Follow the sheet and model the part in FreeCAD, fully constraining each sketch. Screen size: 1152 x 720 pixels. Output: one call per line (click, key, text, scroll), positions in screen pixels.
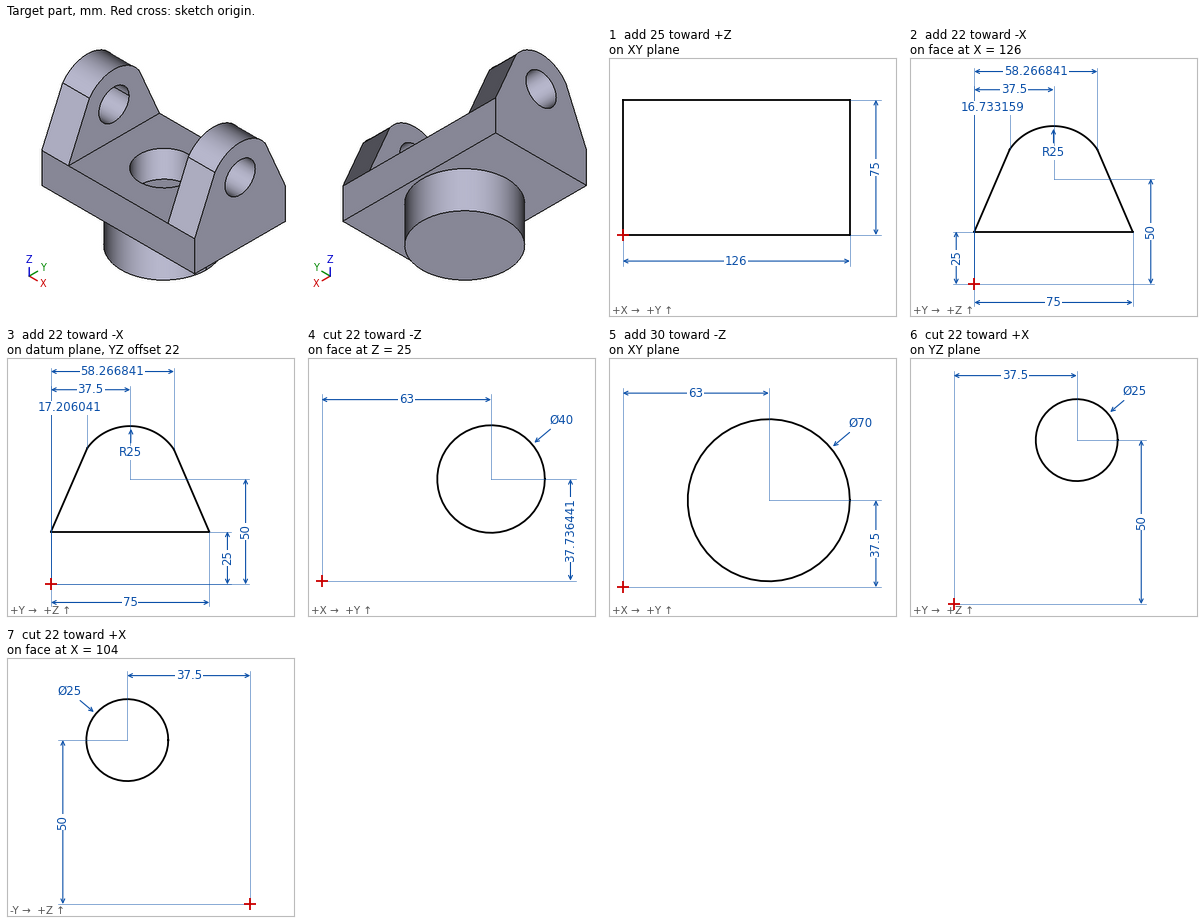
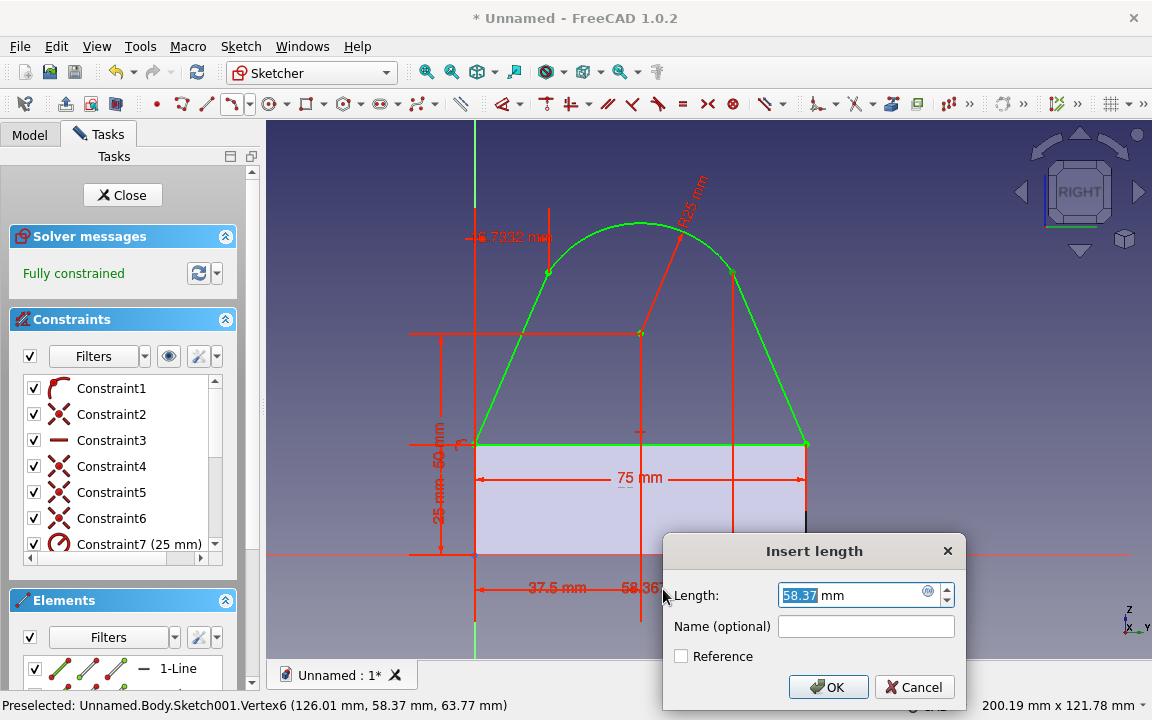
text(58.266841)
key(Return)
key(Escape)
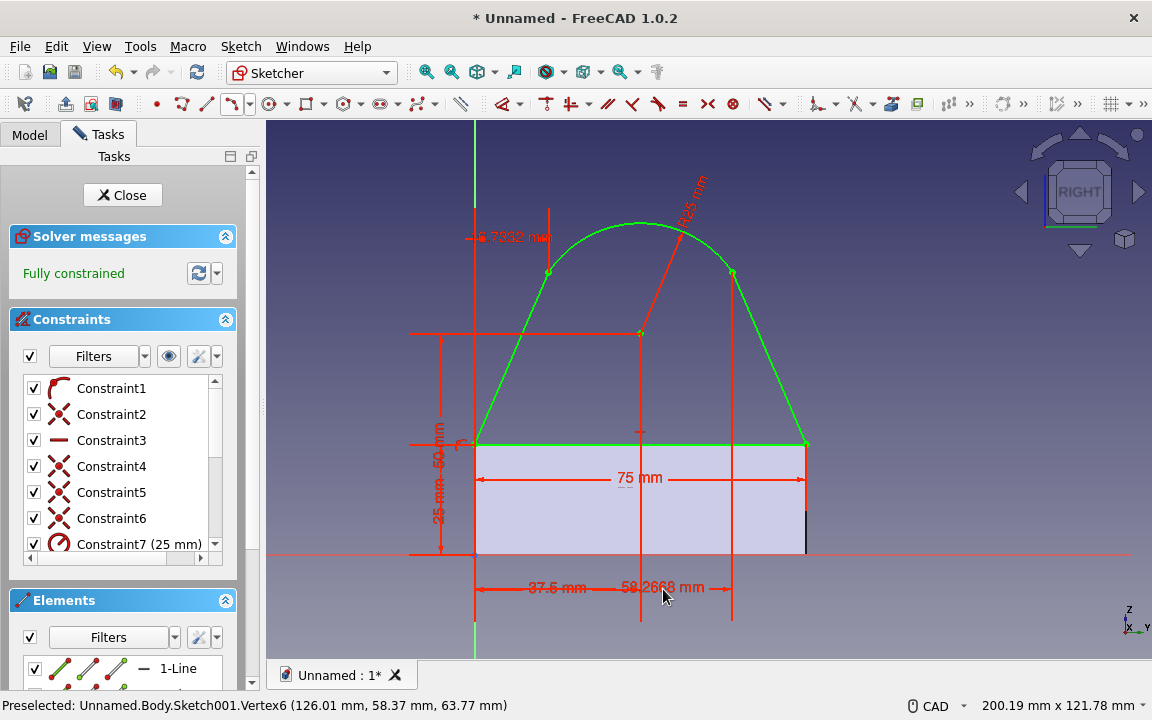
click(123, 195)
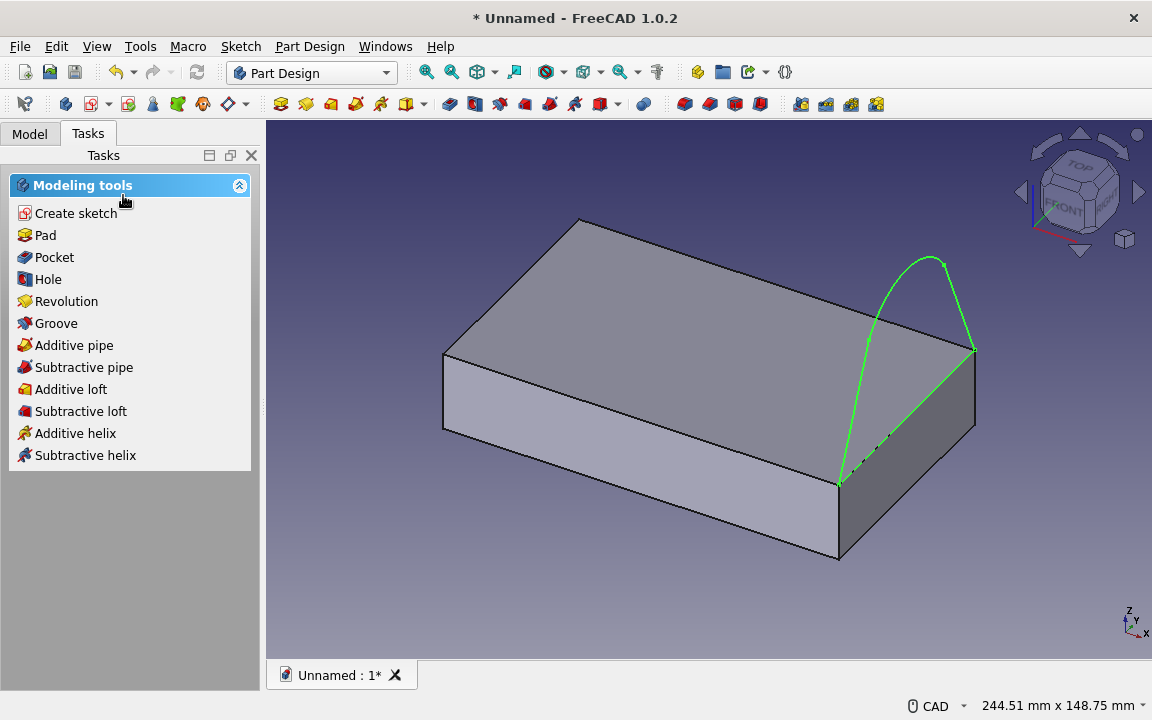
click(281, 104)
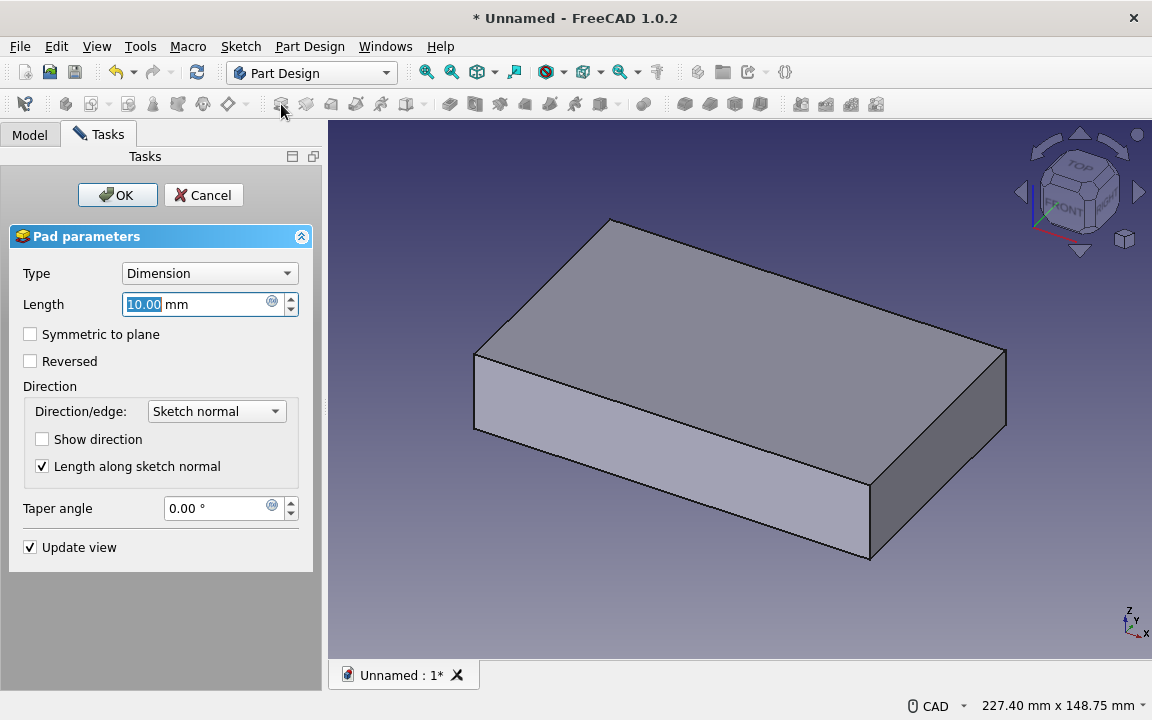
text(22)
key(Tab)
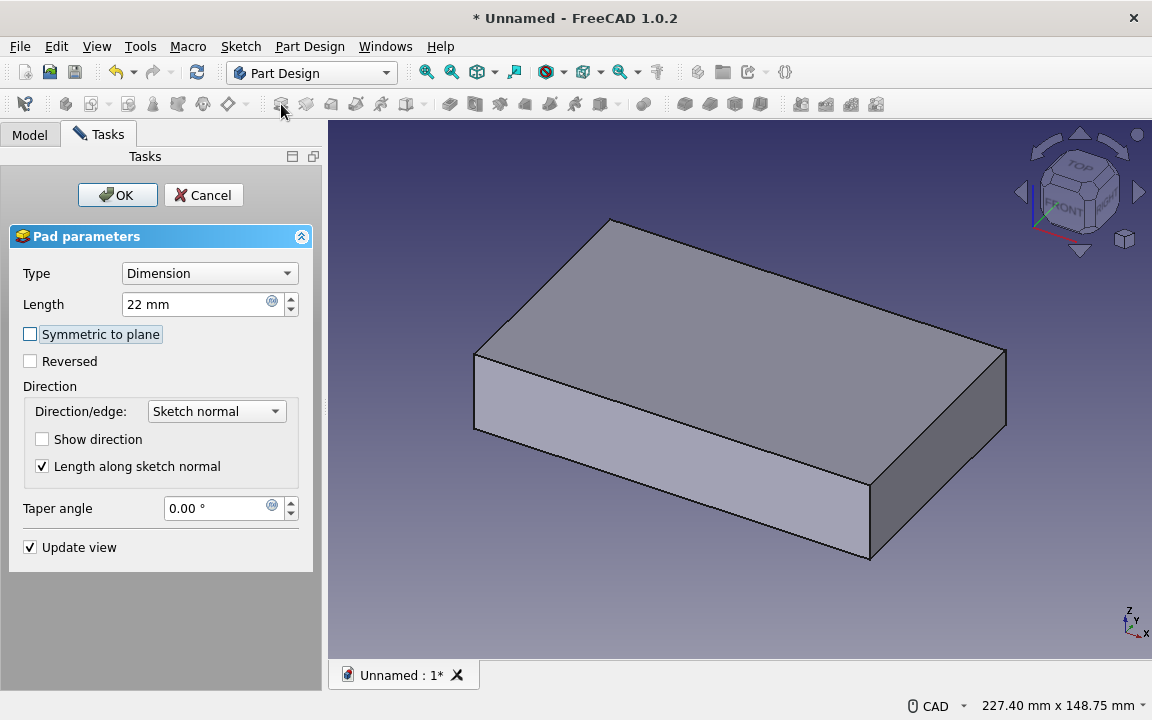
click(31, 361)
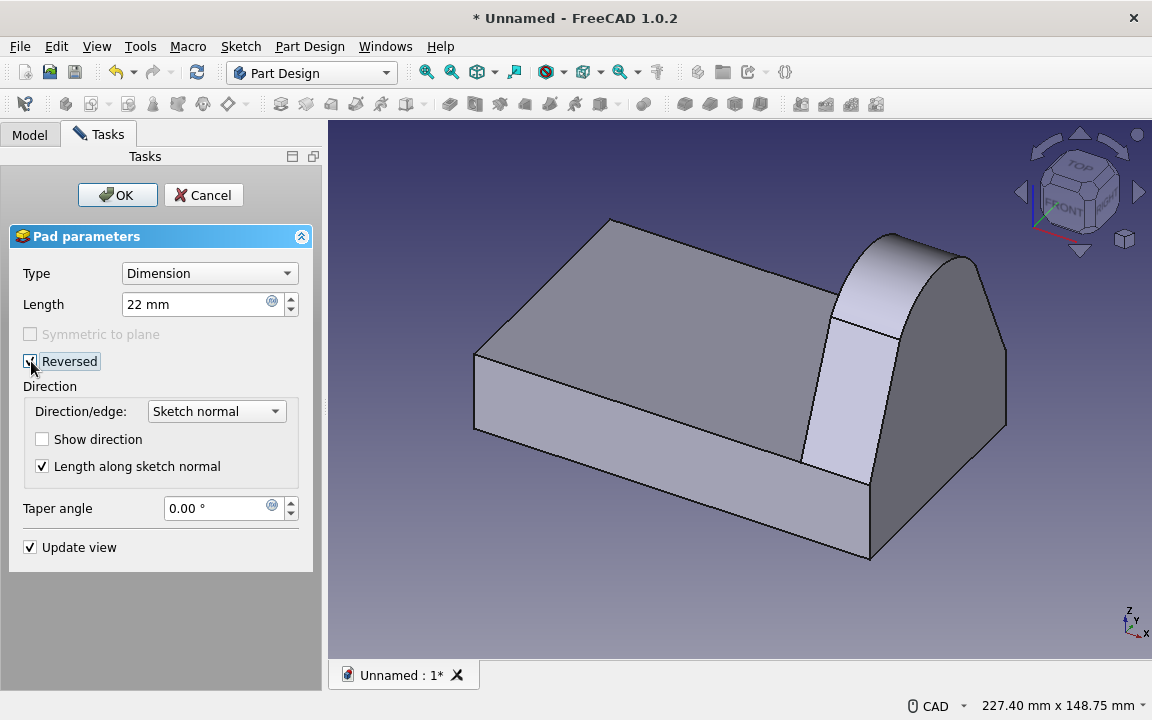
click(118, 195)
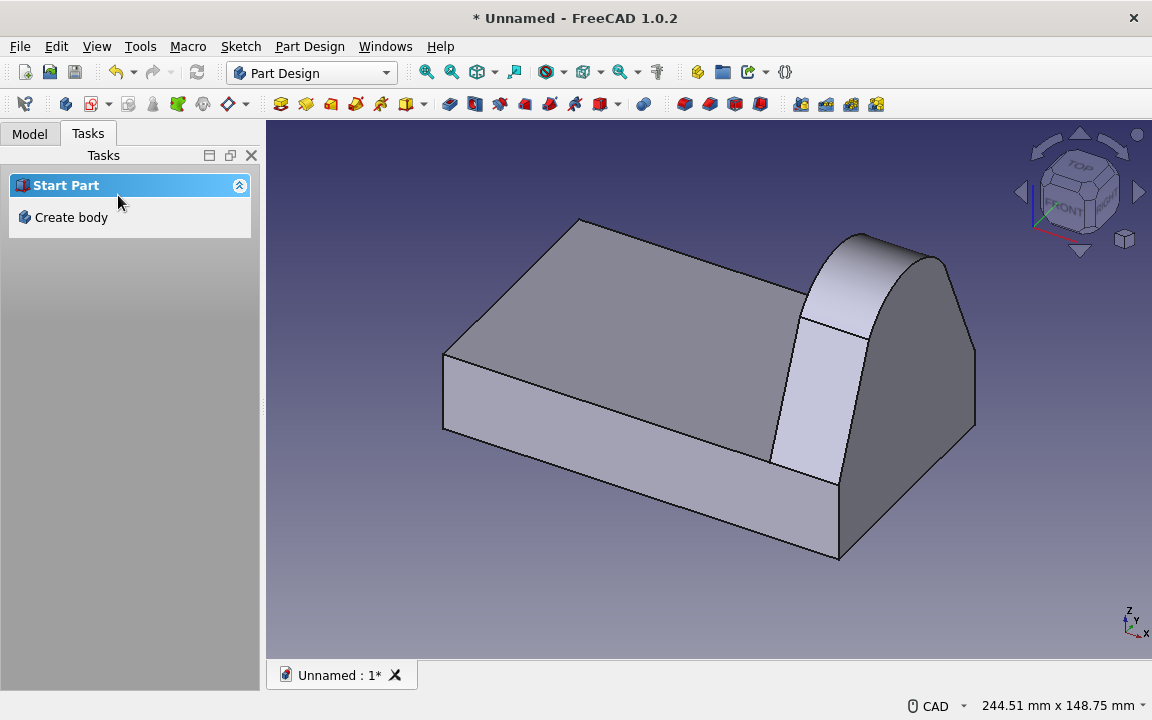
click(427, 72)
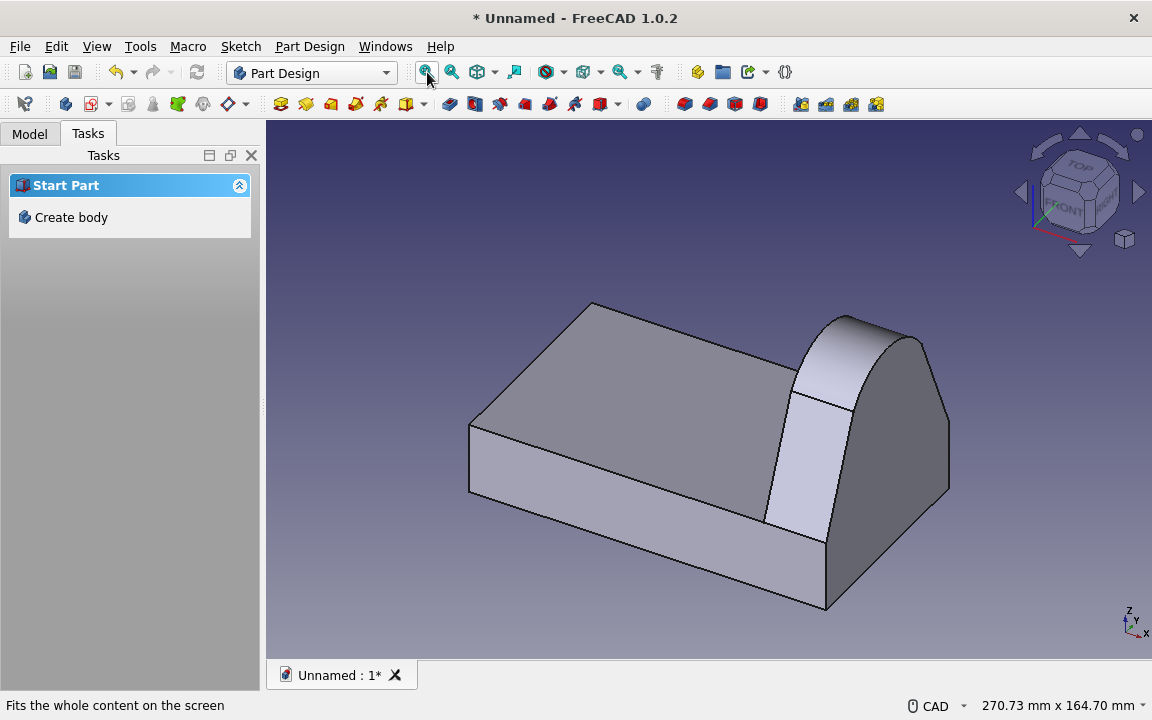
click(30, 134)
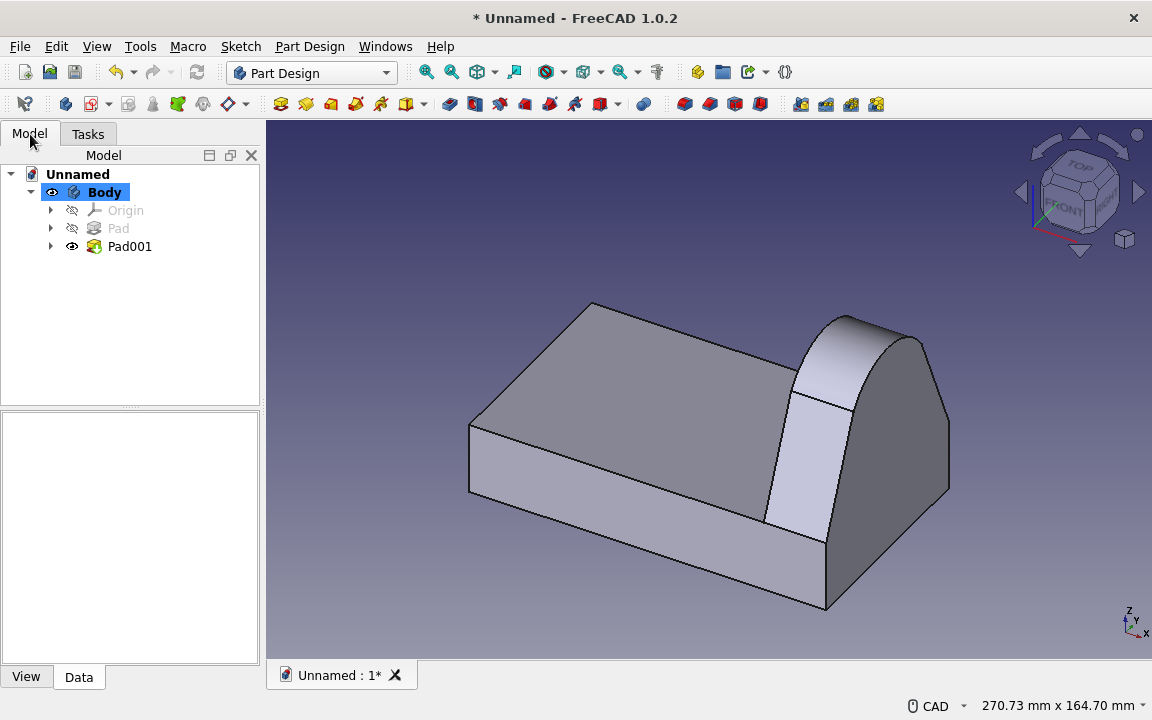
click(51, 210)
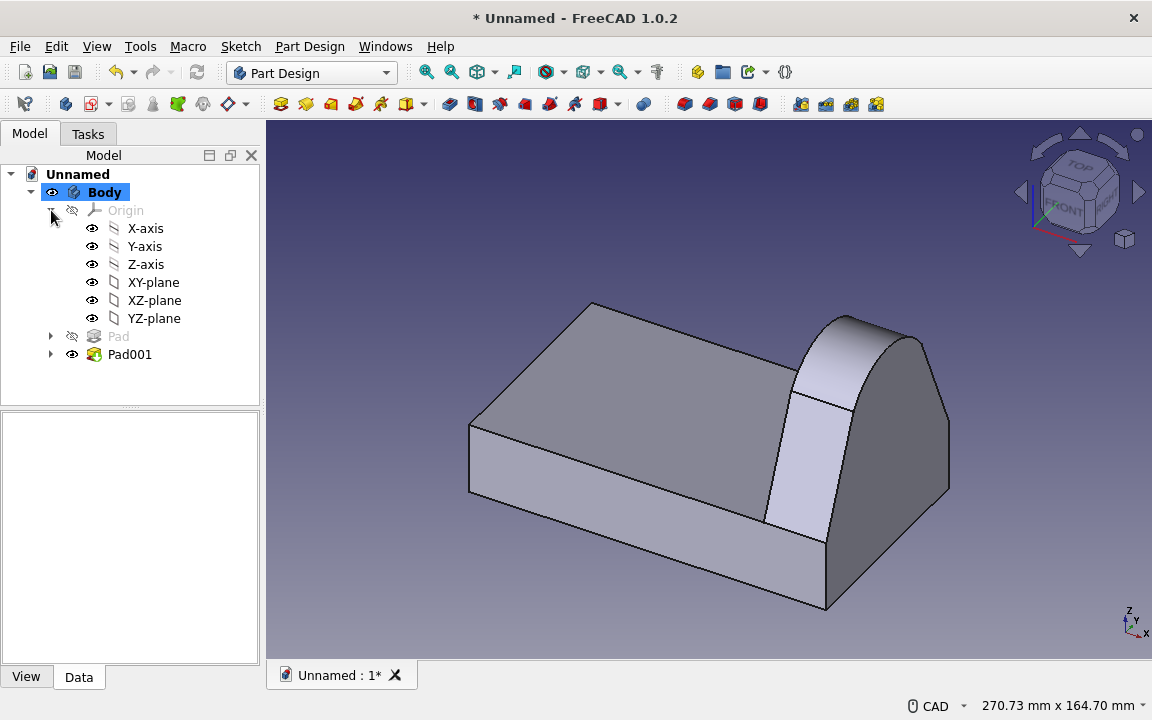
click(137, 318)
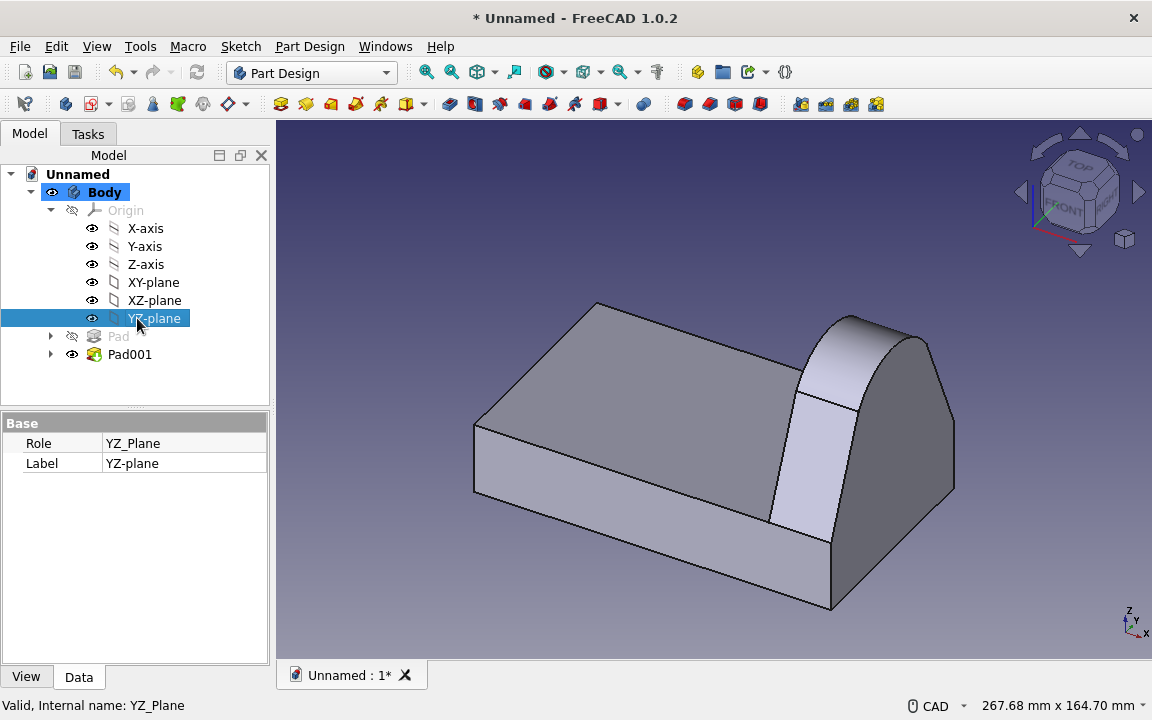
click(228, 104)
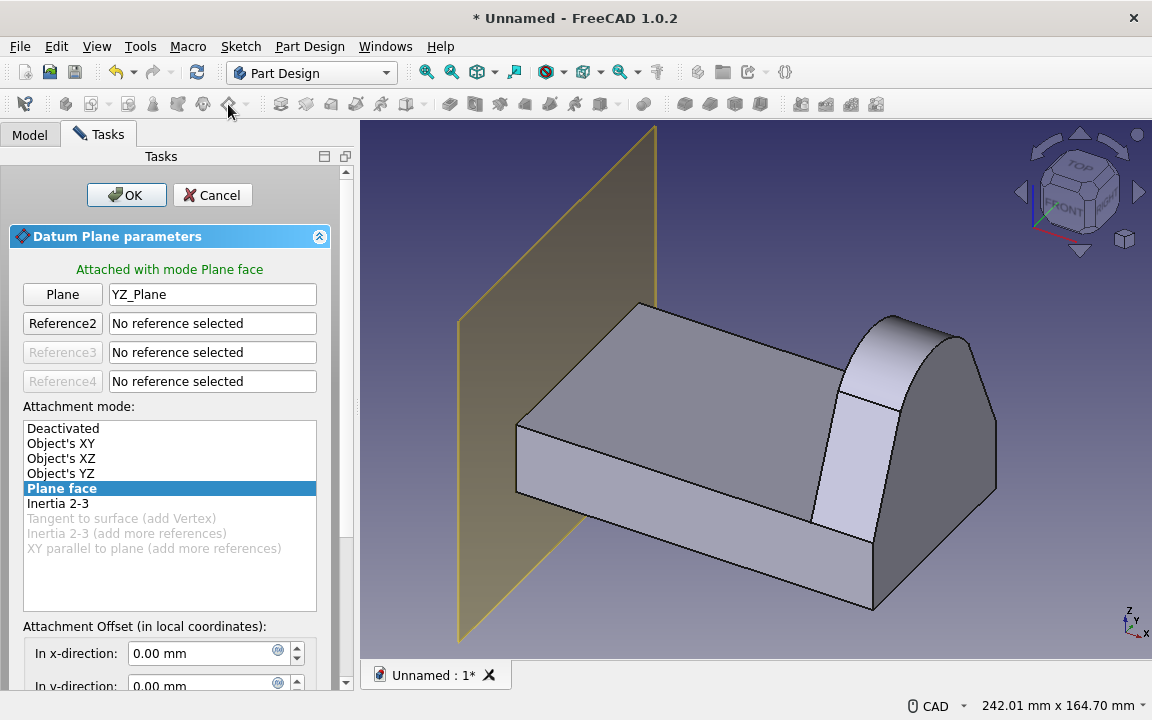
scroll(346, 428, down, 2)